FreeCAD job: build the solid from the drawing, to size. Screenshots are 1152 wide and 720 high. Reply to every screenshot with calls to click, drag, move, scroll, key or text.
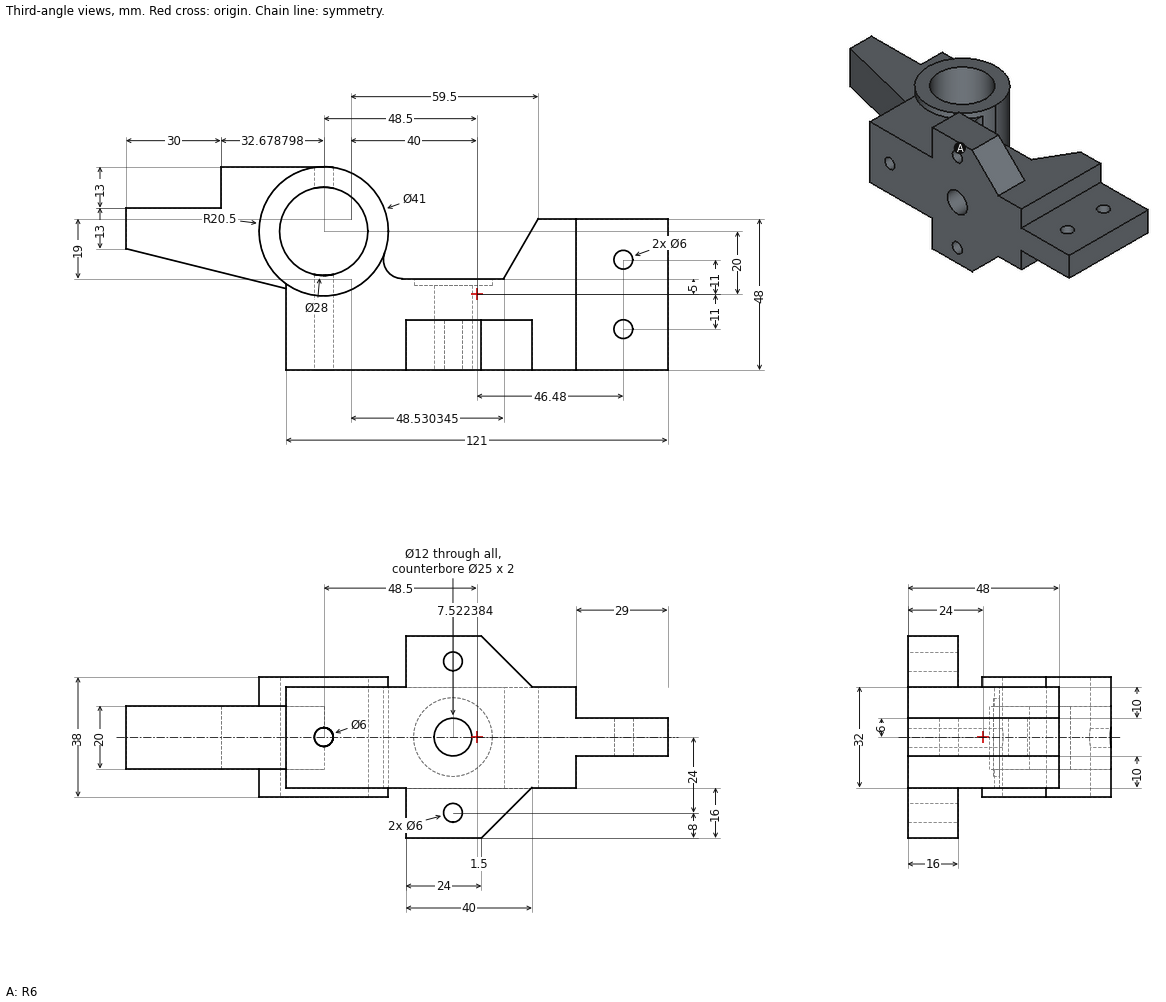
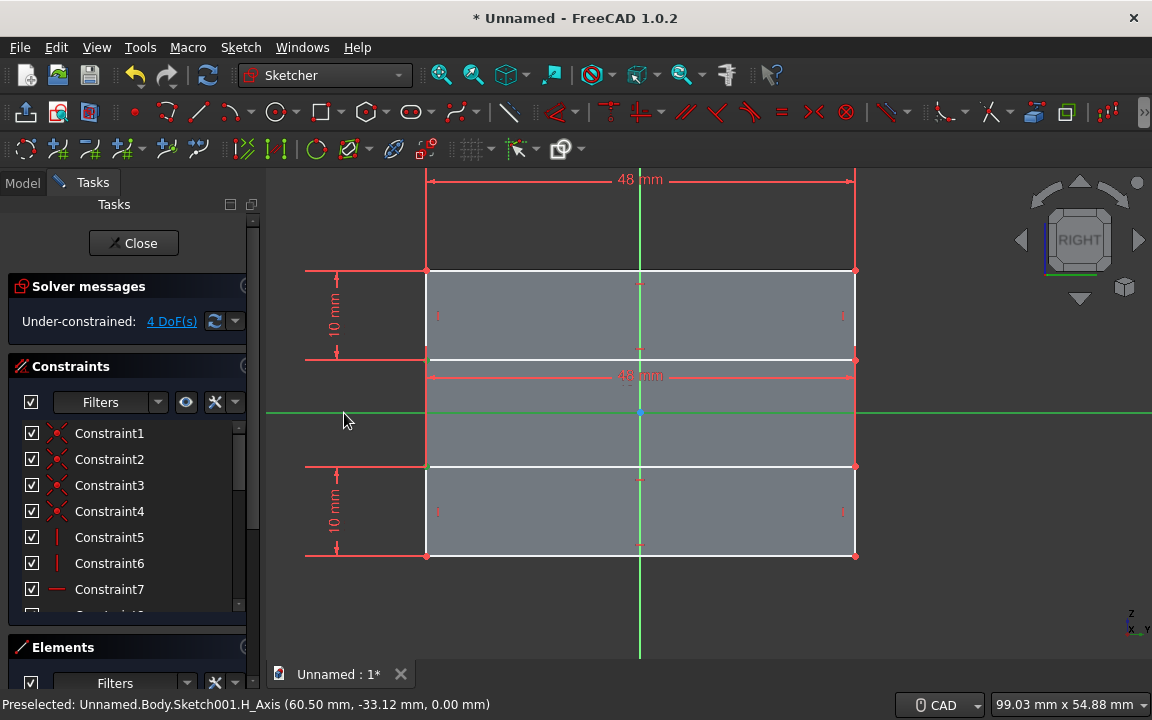
click(814, 112)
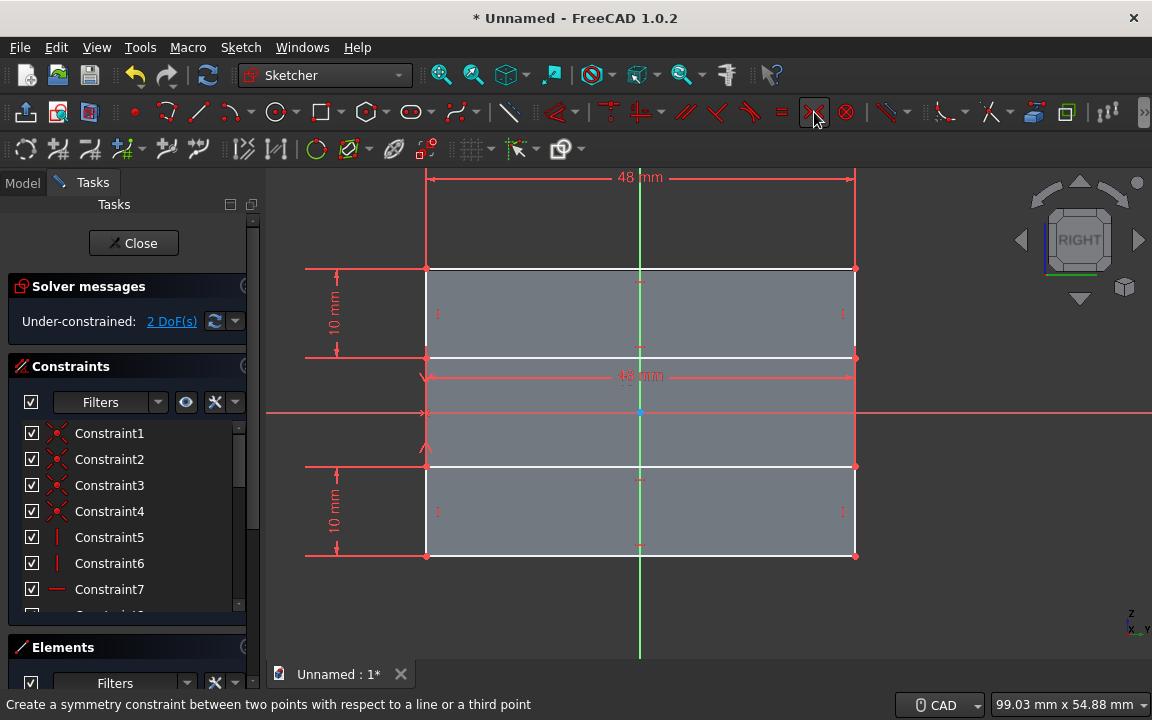
click(426, 358)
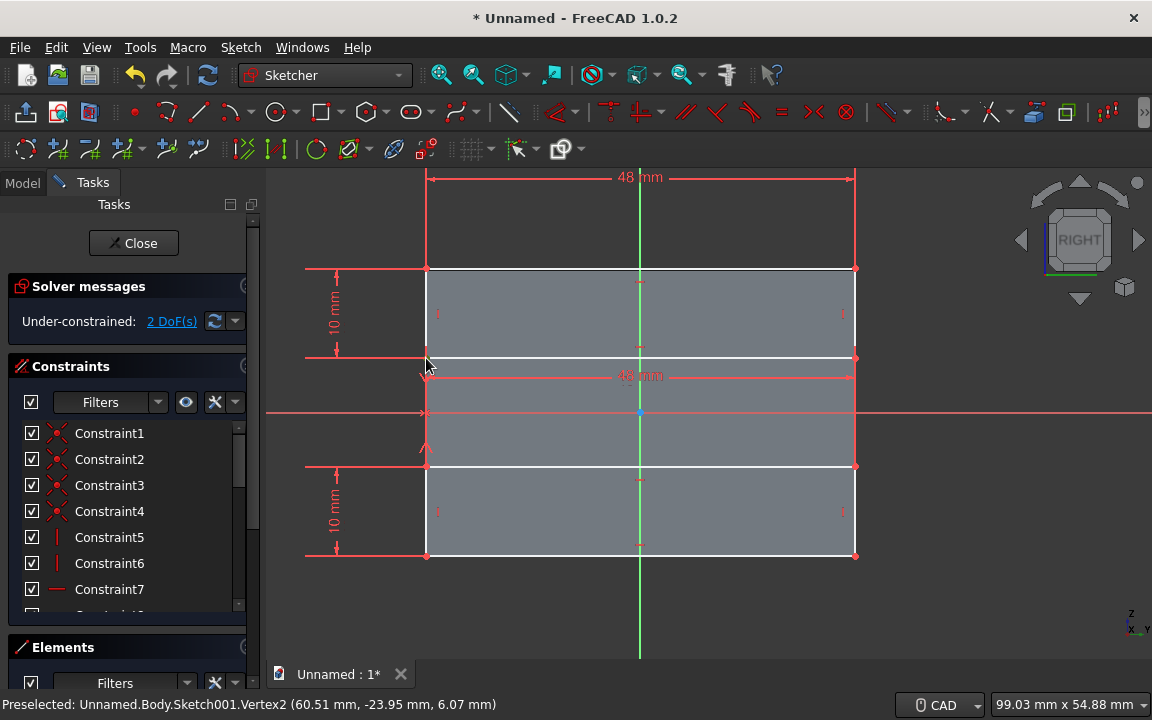
key(i)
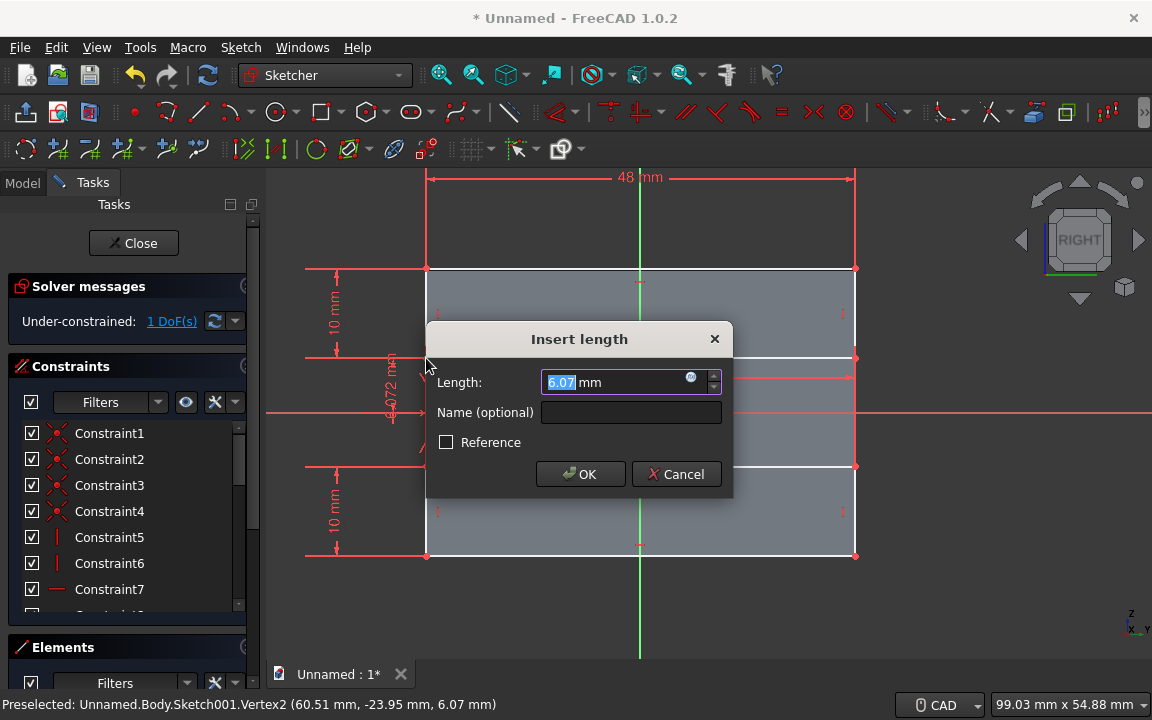
text(6)
key(Return)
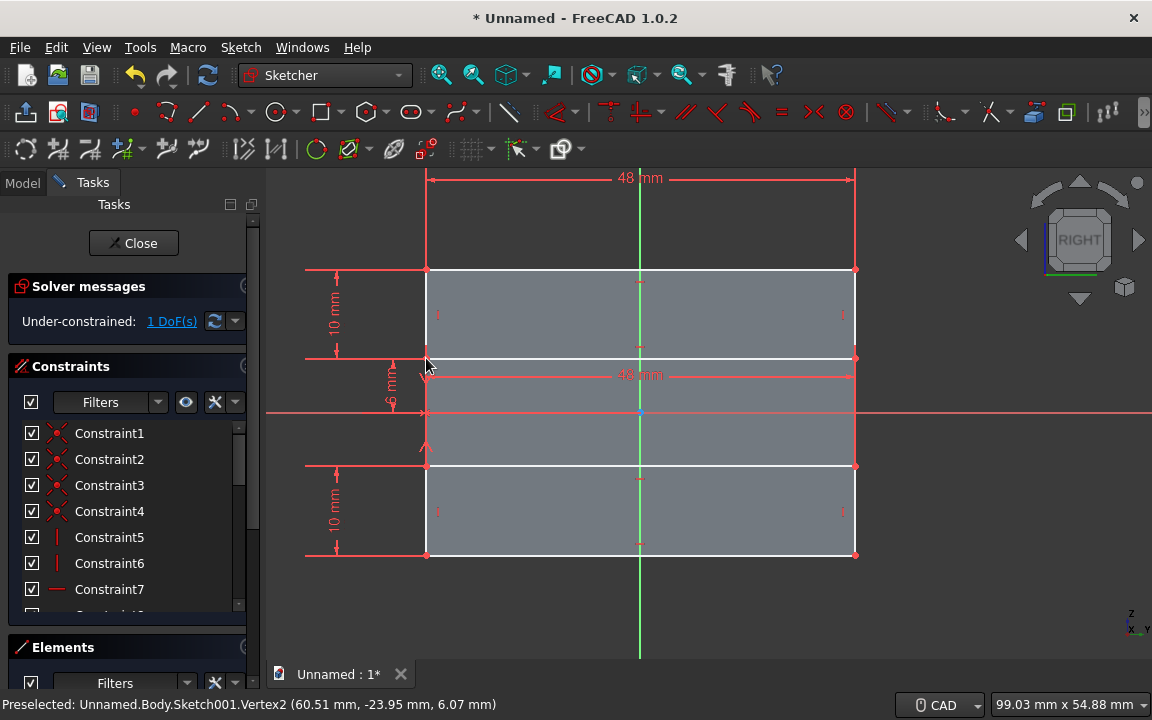
click(426, 270)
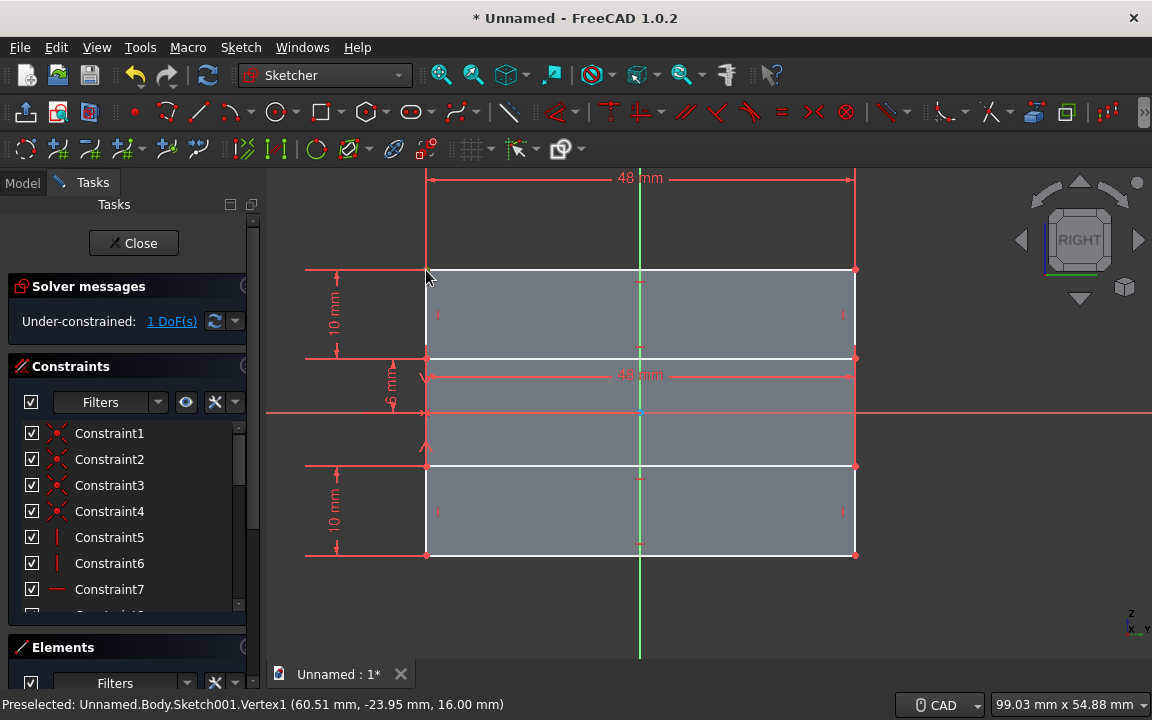
key(l)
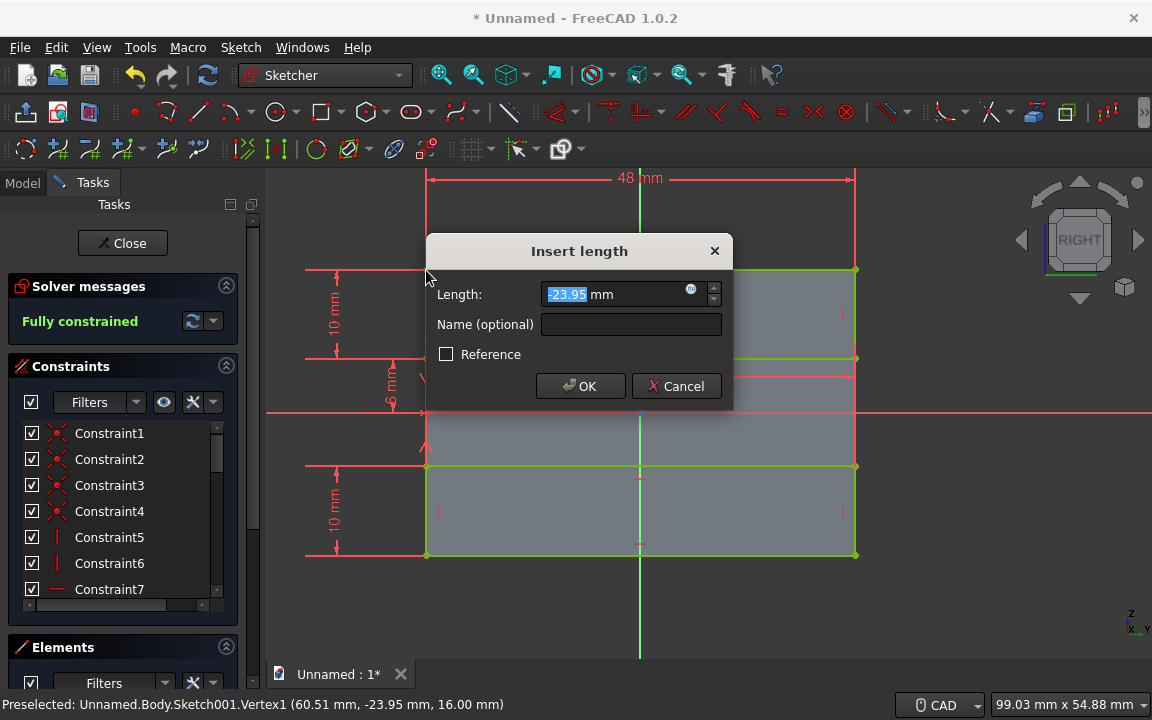
text(-24)
key(Return)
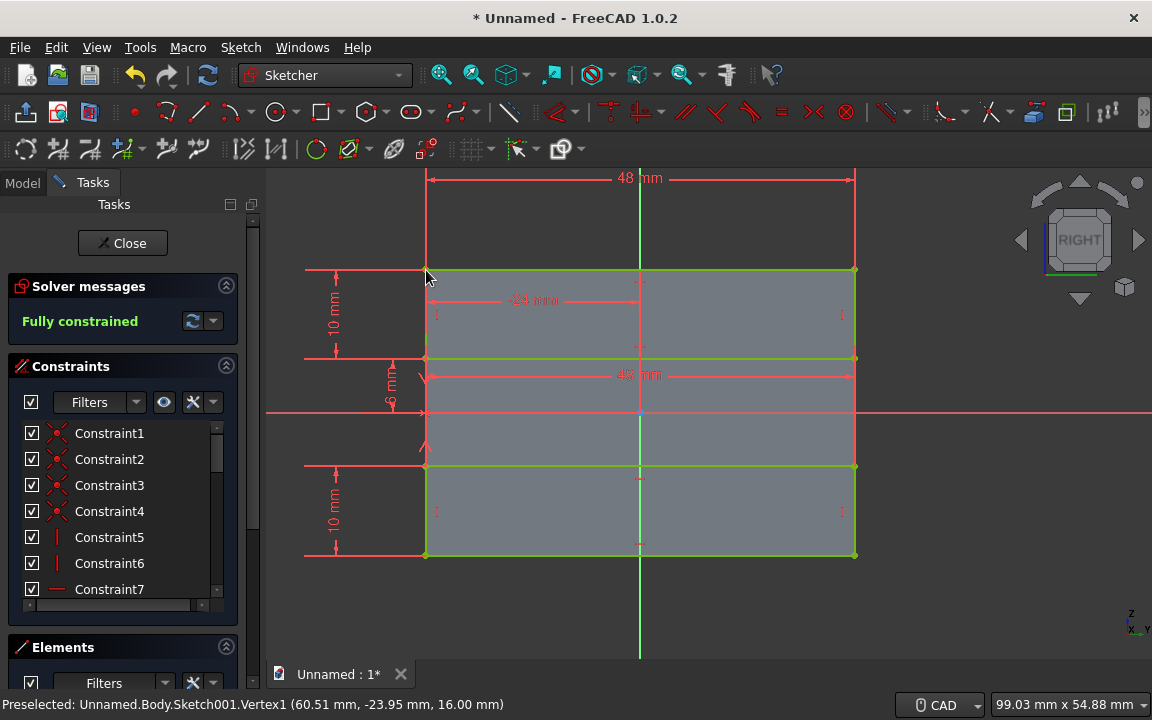
click(123, 243)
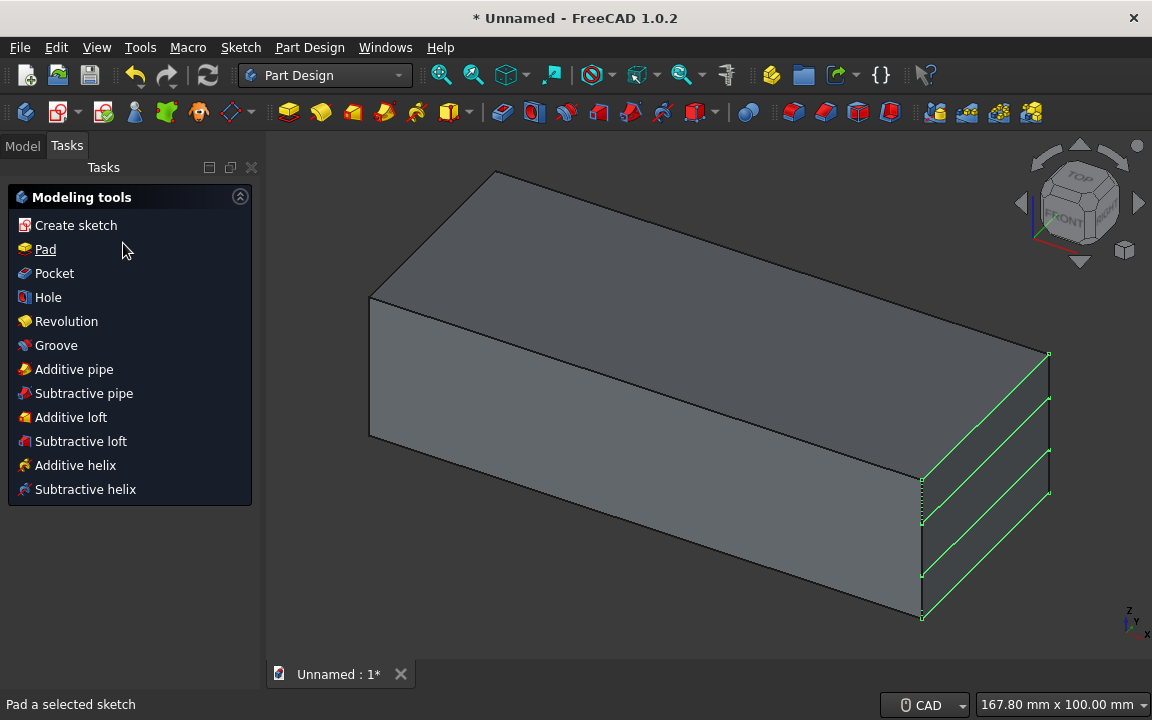
click(504, 112)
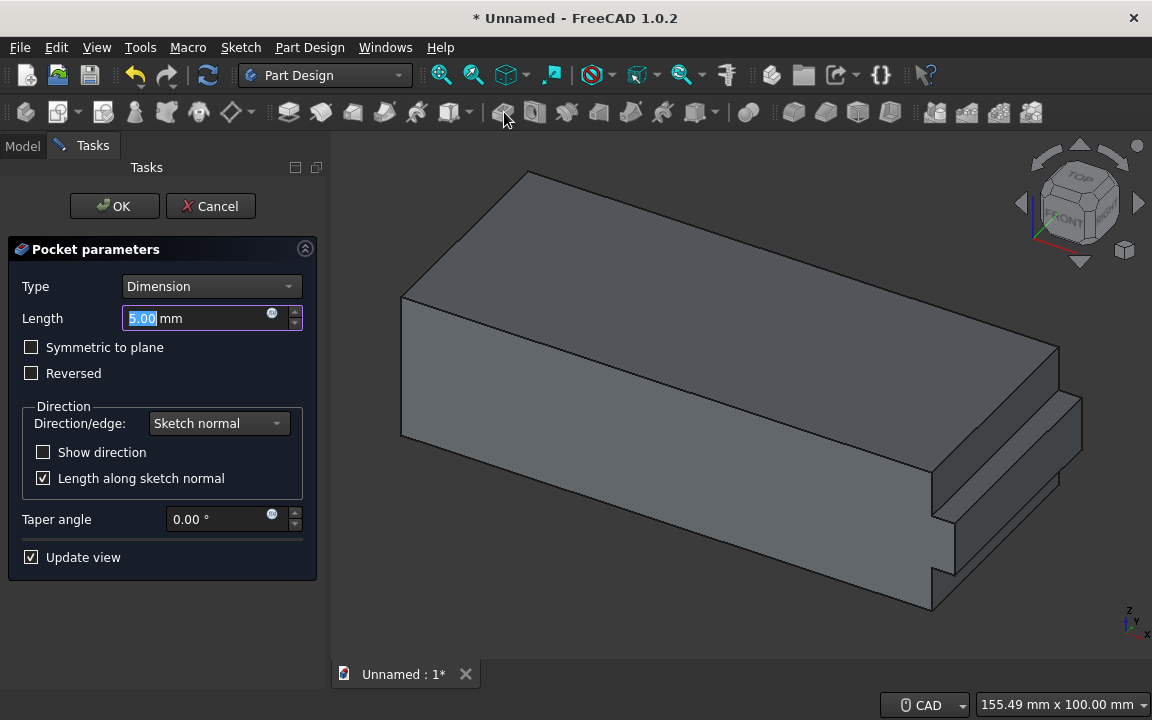
text(29)
key(Tab)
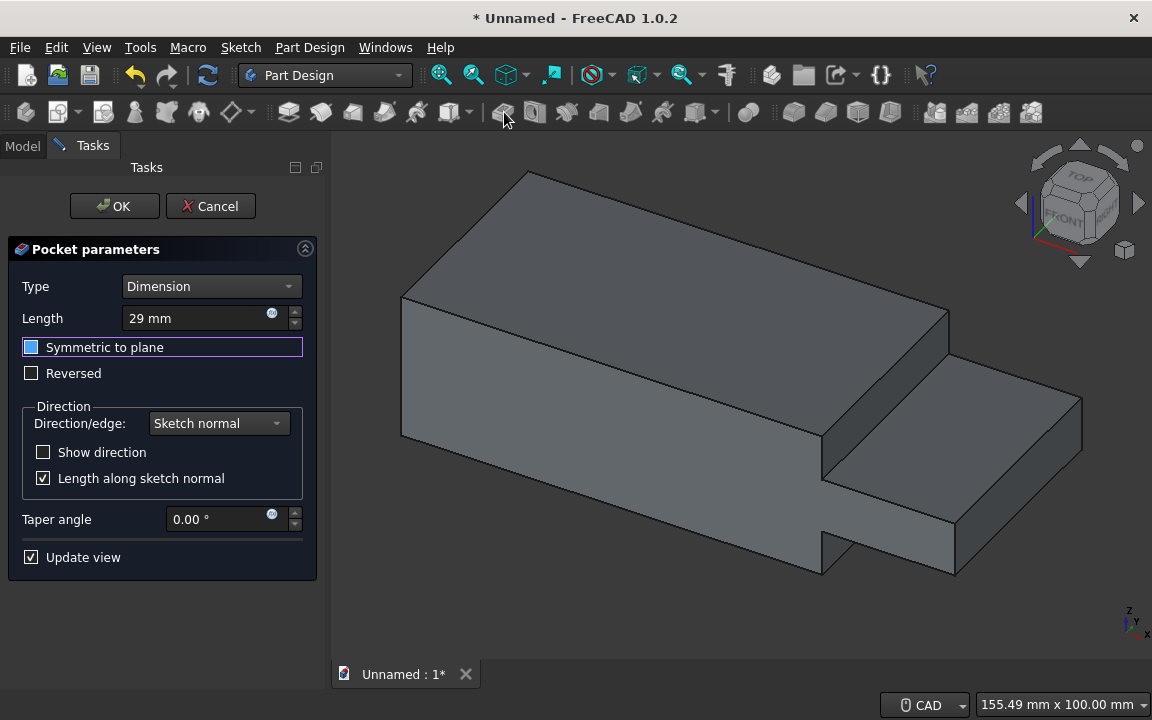
click(115, 206)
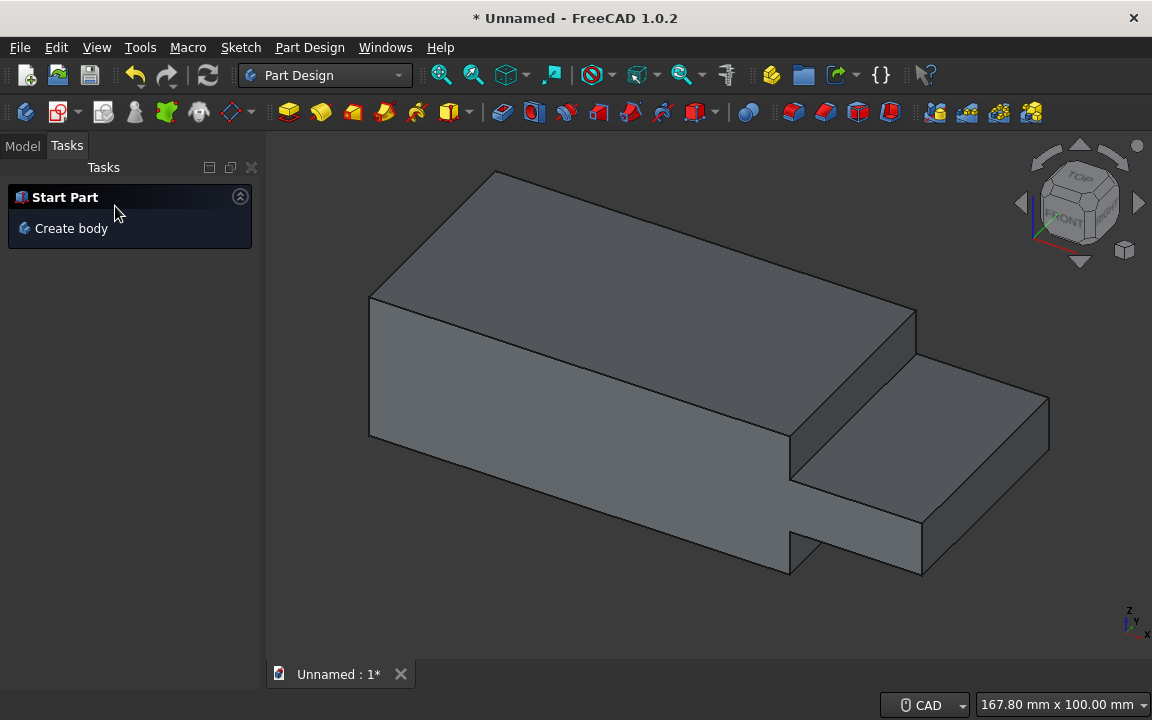
click(703, 323)